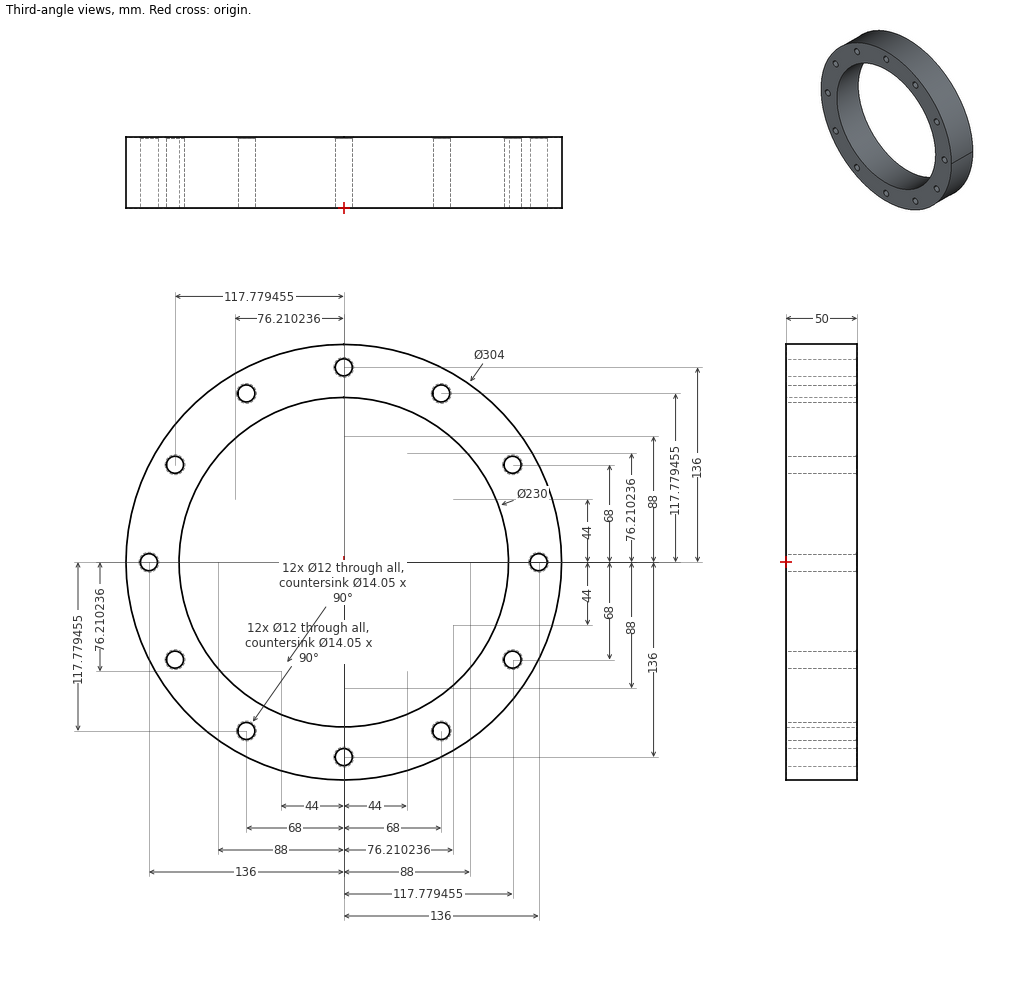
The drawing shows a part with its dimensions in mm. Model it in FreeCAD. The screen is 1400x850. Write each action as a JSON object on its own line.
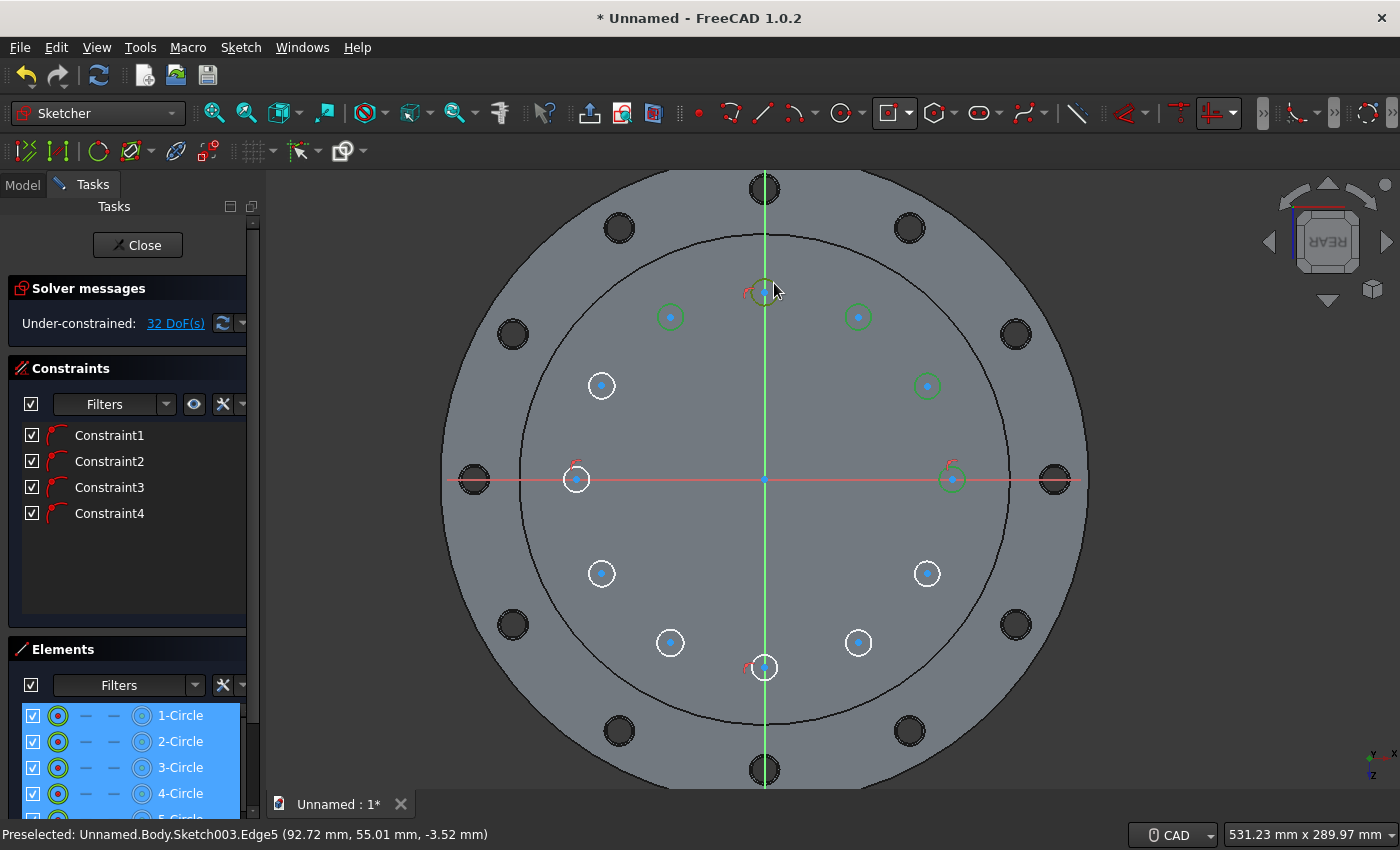
{"action": "left_click", "coordinate": [936, 565]}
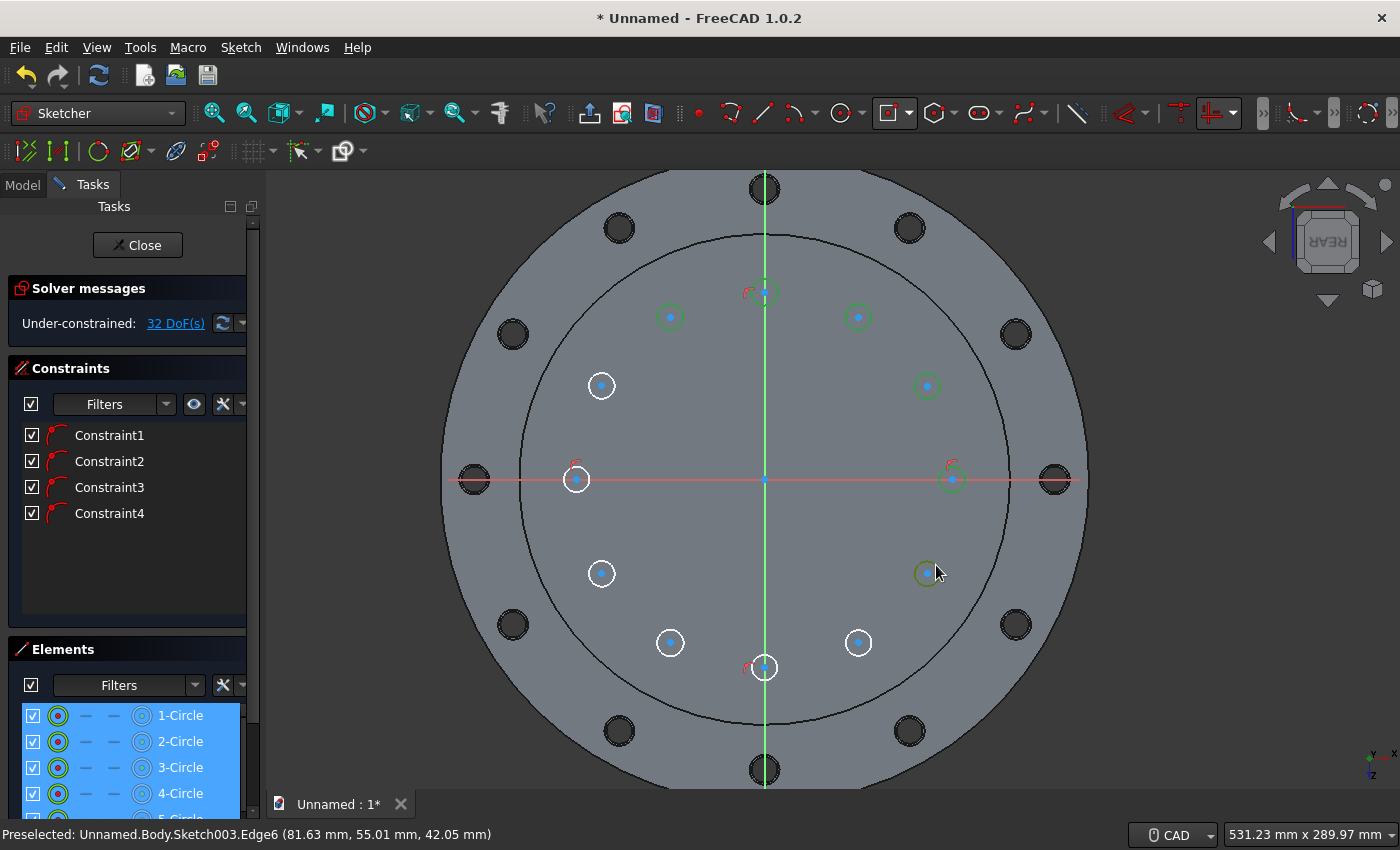
{"action": "left_click", "coordinate": [868, 634]}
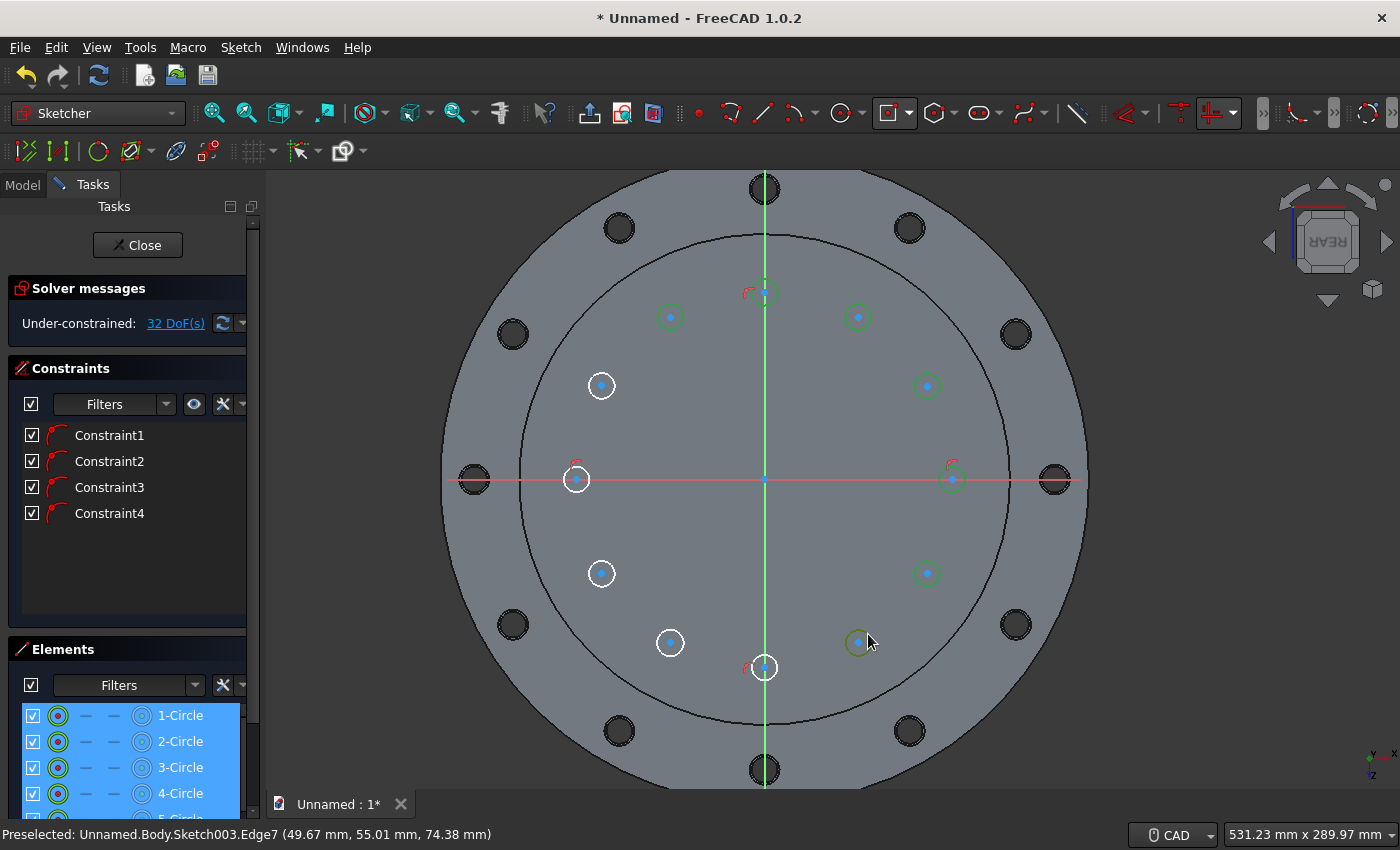
{"action": "left_click", "coordinate": [765, 655]}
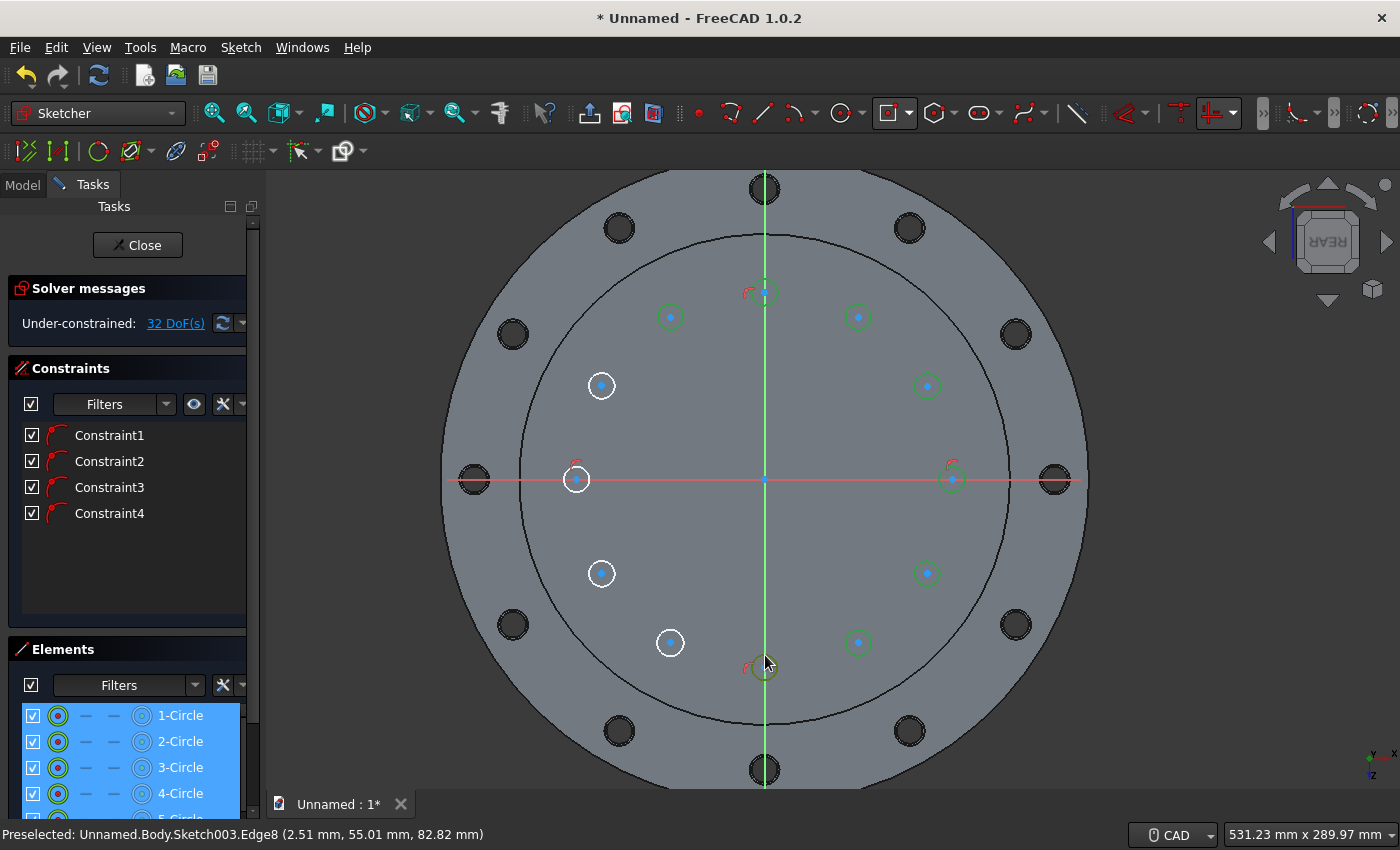
{"action": "left_click", "coordinate": [680, 634]}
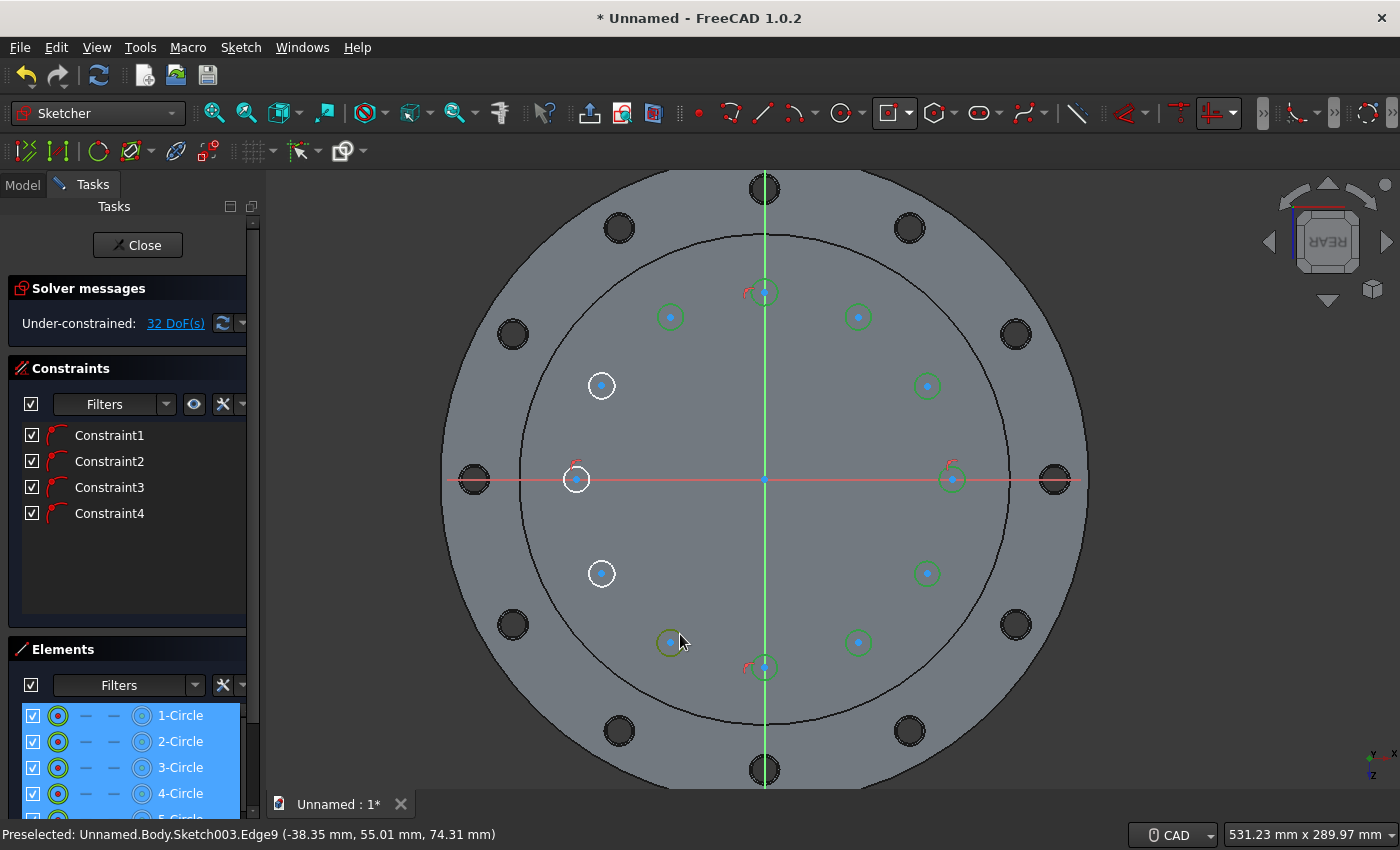
{"action": "left_click", "coordinate": [611, 565]}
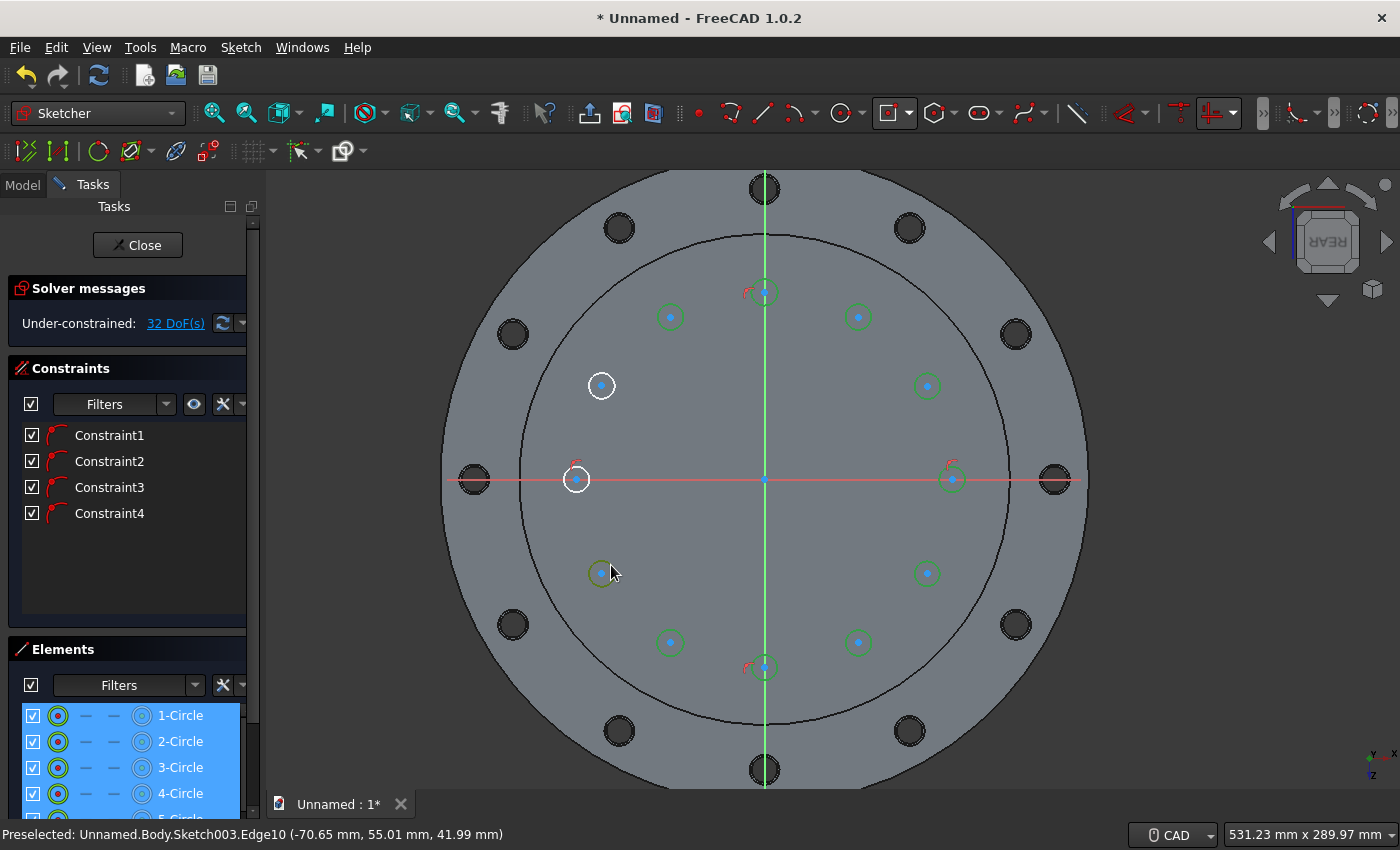
{"action": "left_click", "coordinate": [564, 479]}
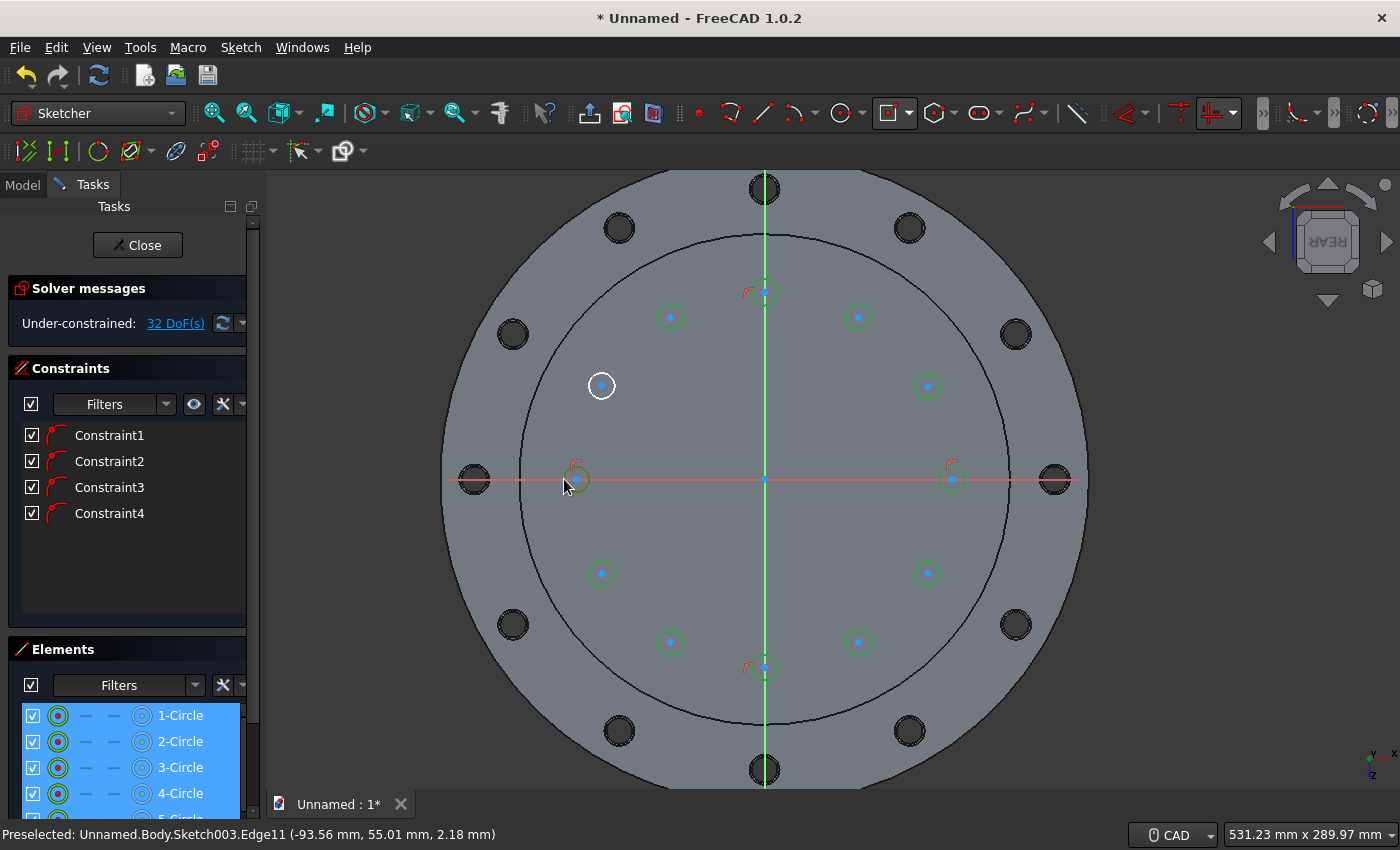
{"action": "left_click", "coordinate": [611, 377]}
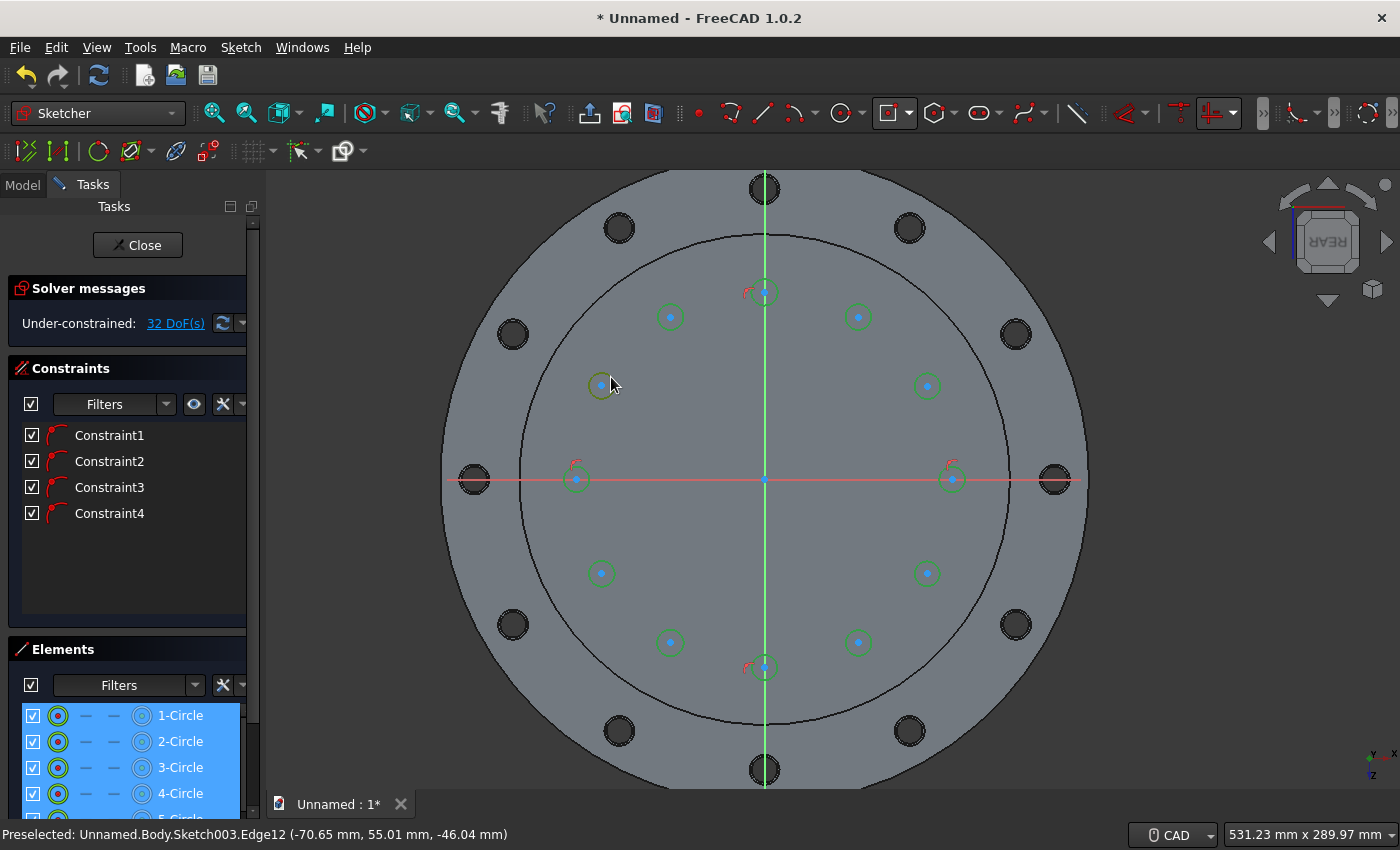
{"action": "key", "text": "e"}